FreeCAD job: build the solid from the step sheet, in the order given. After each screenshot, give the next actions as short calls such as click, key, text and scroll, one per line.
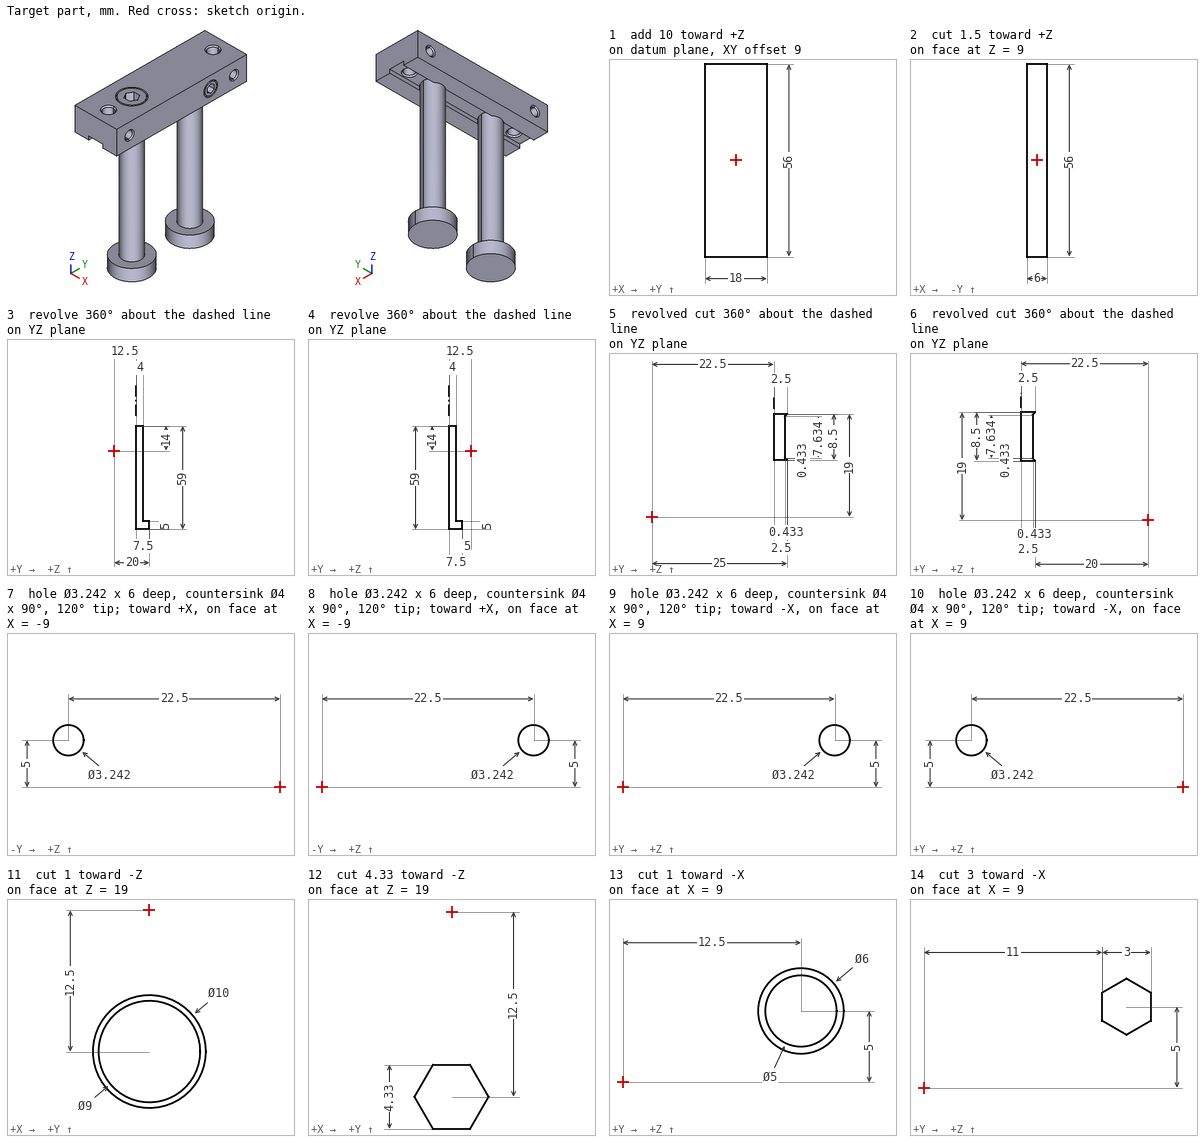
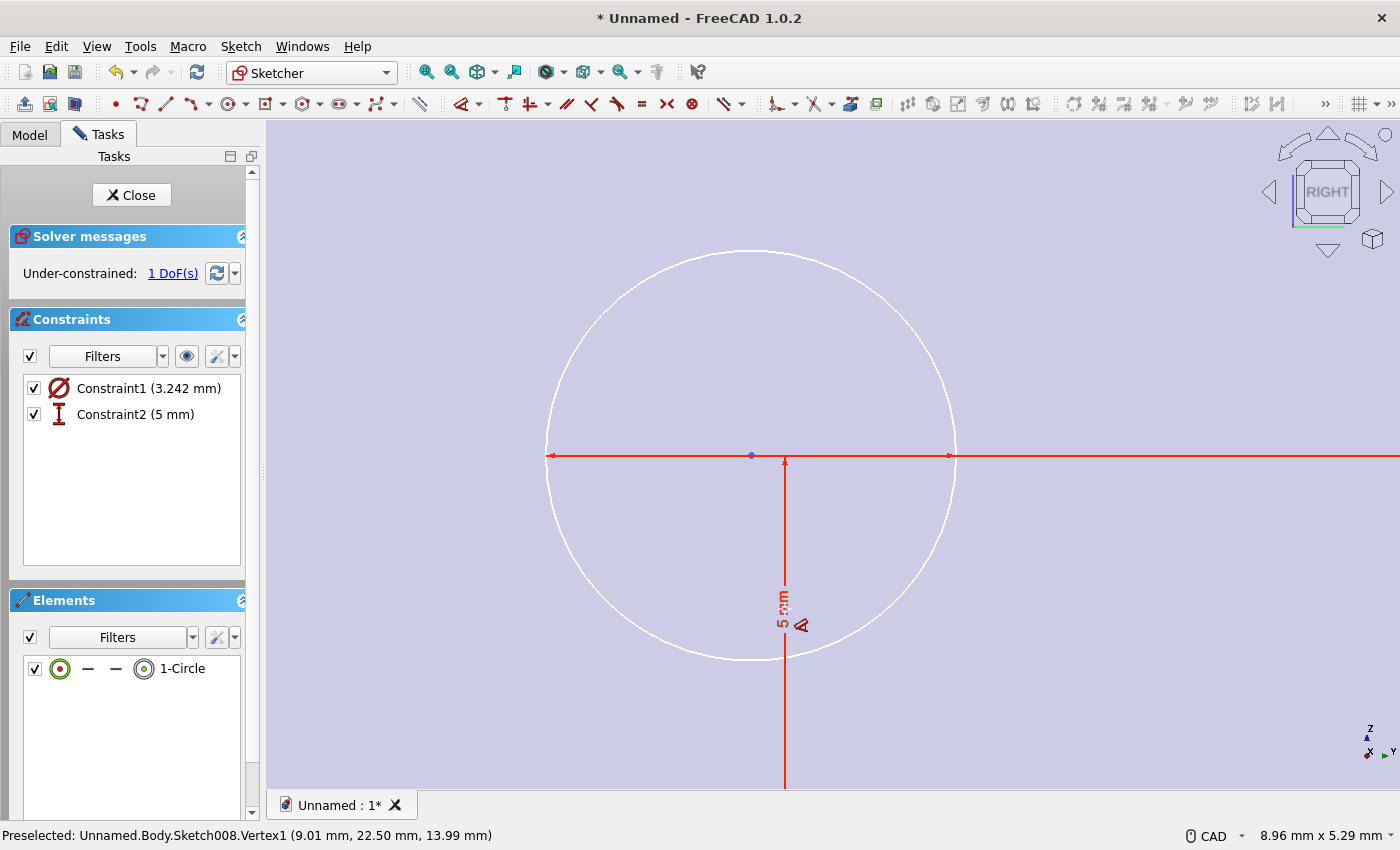
click(751, 456)
click(523, 422)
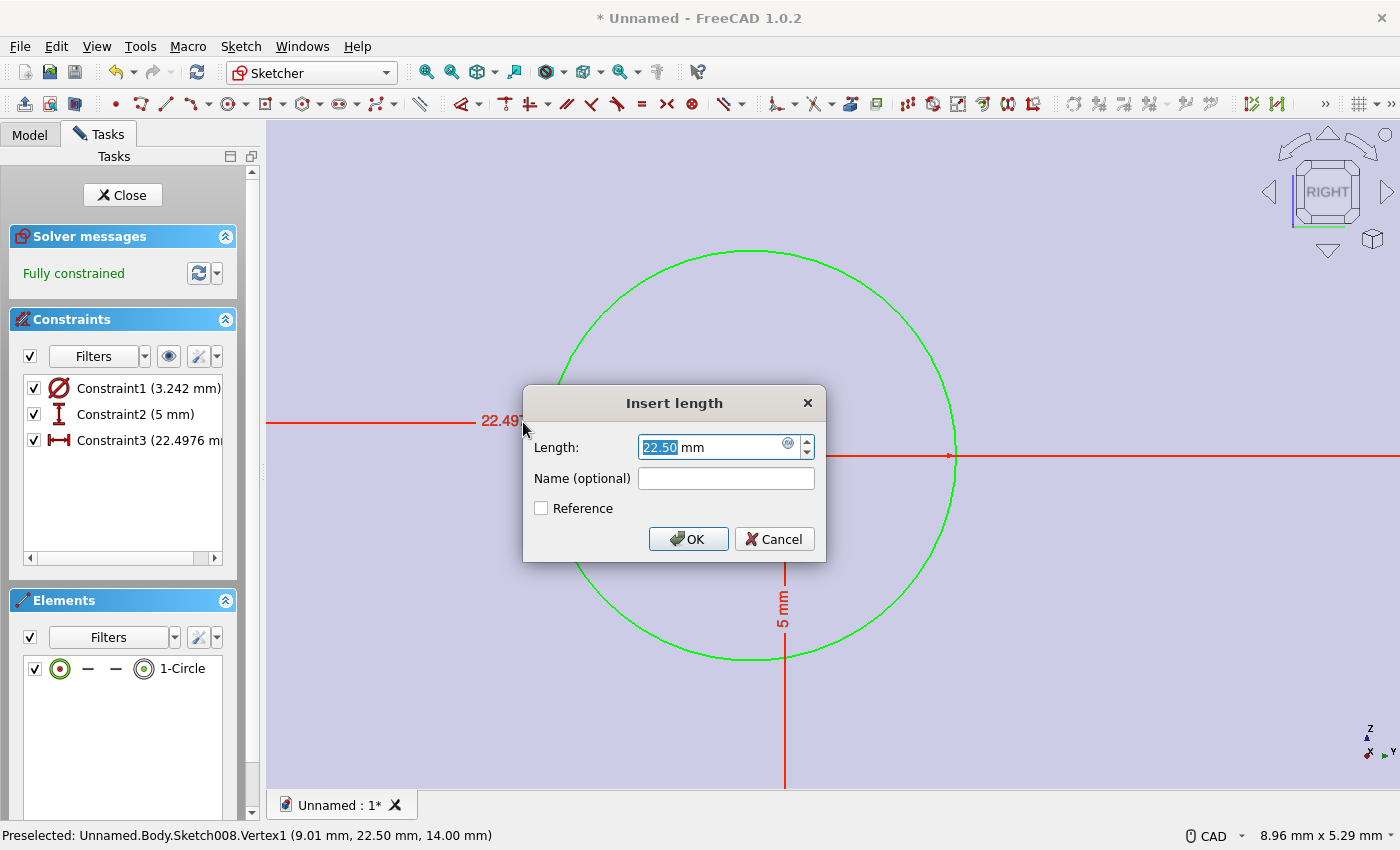
text(22.5)
key(Return)
key(Escape)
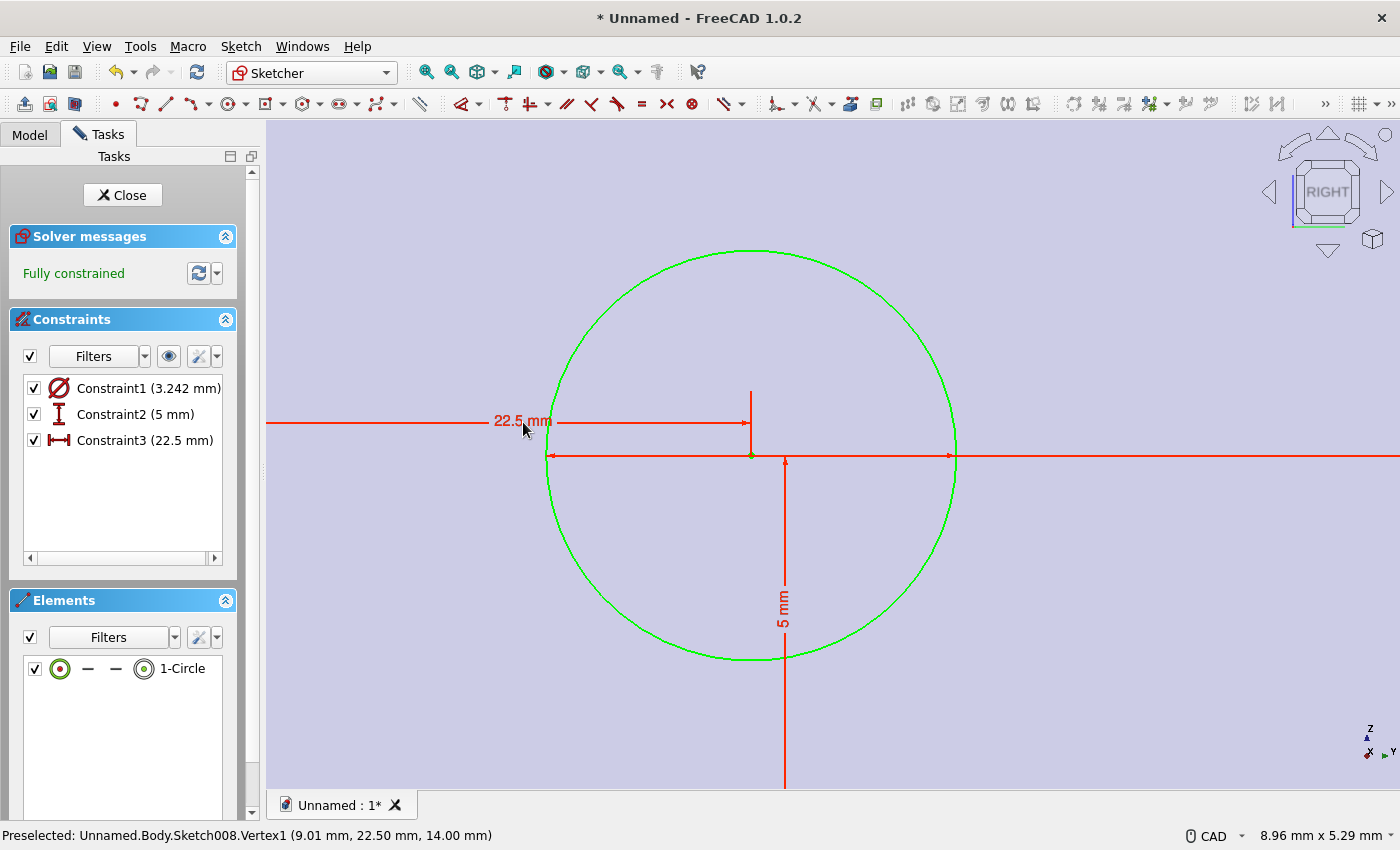
click(123, 195)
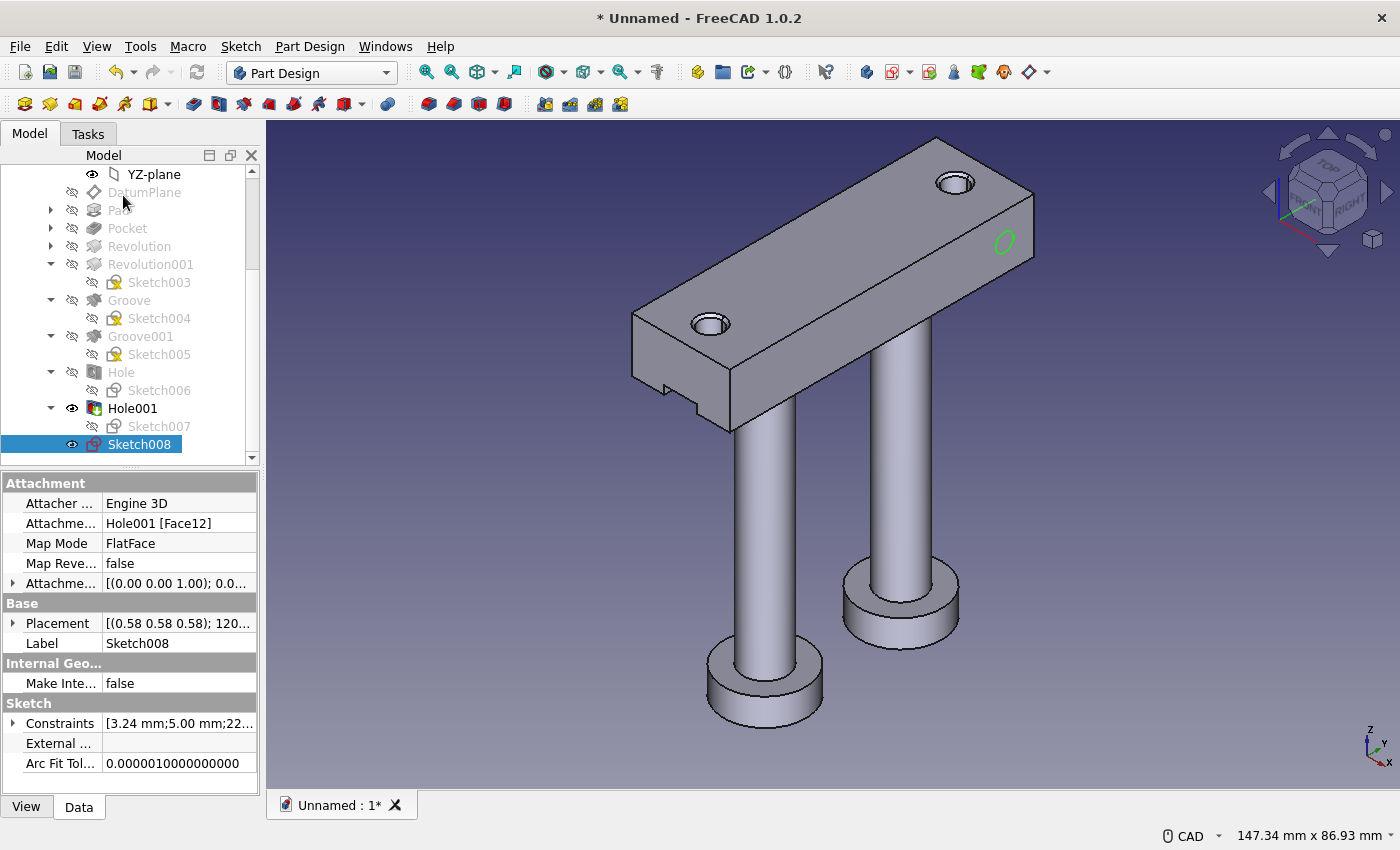
click(219, 104)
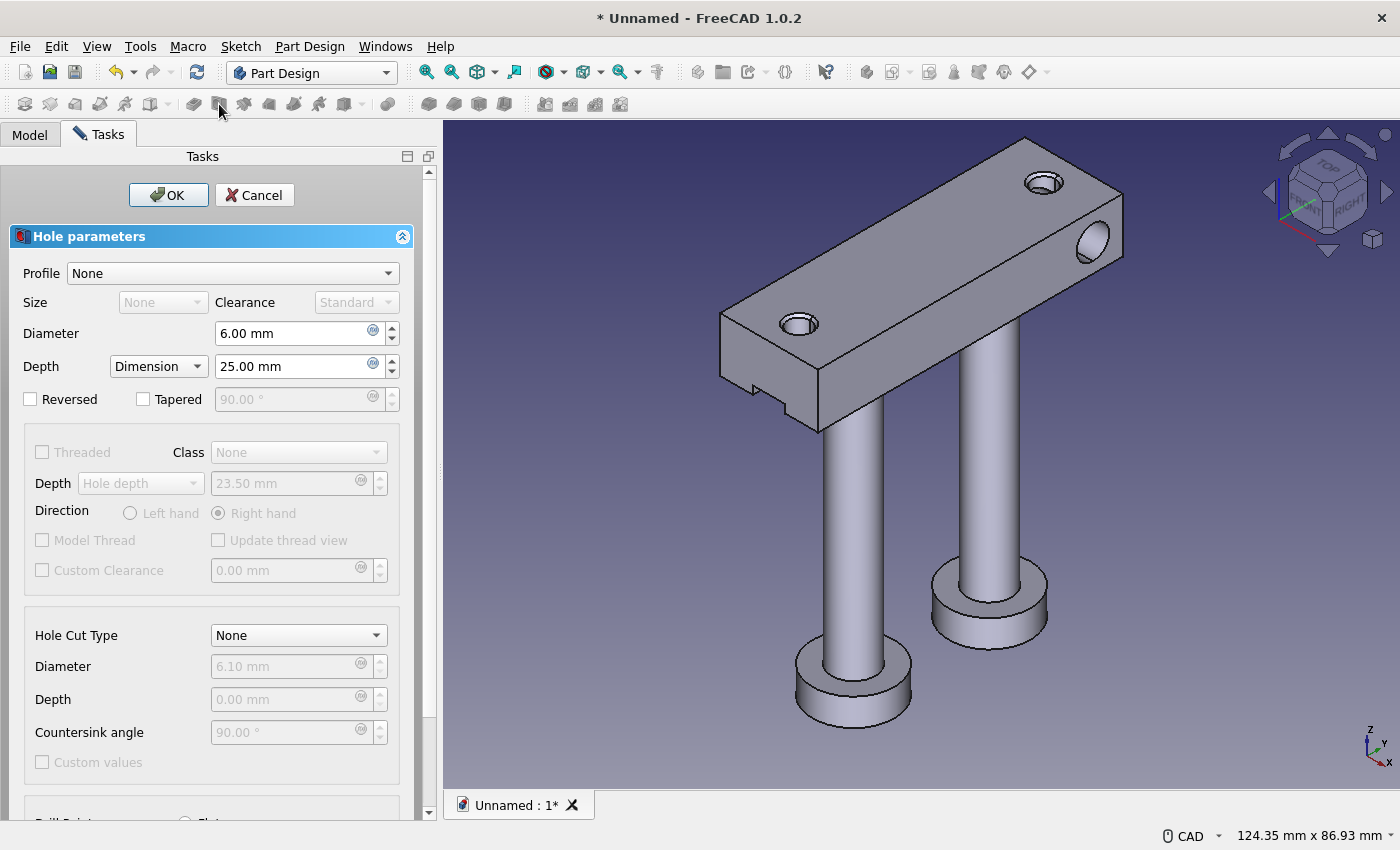
triple_click(300, 334)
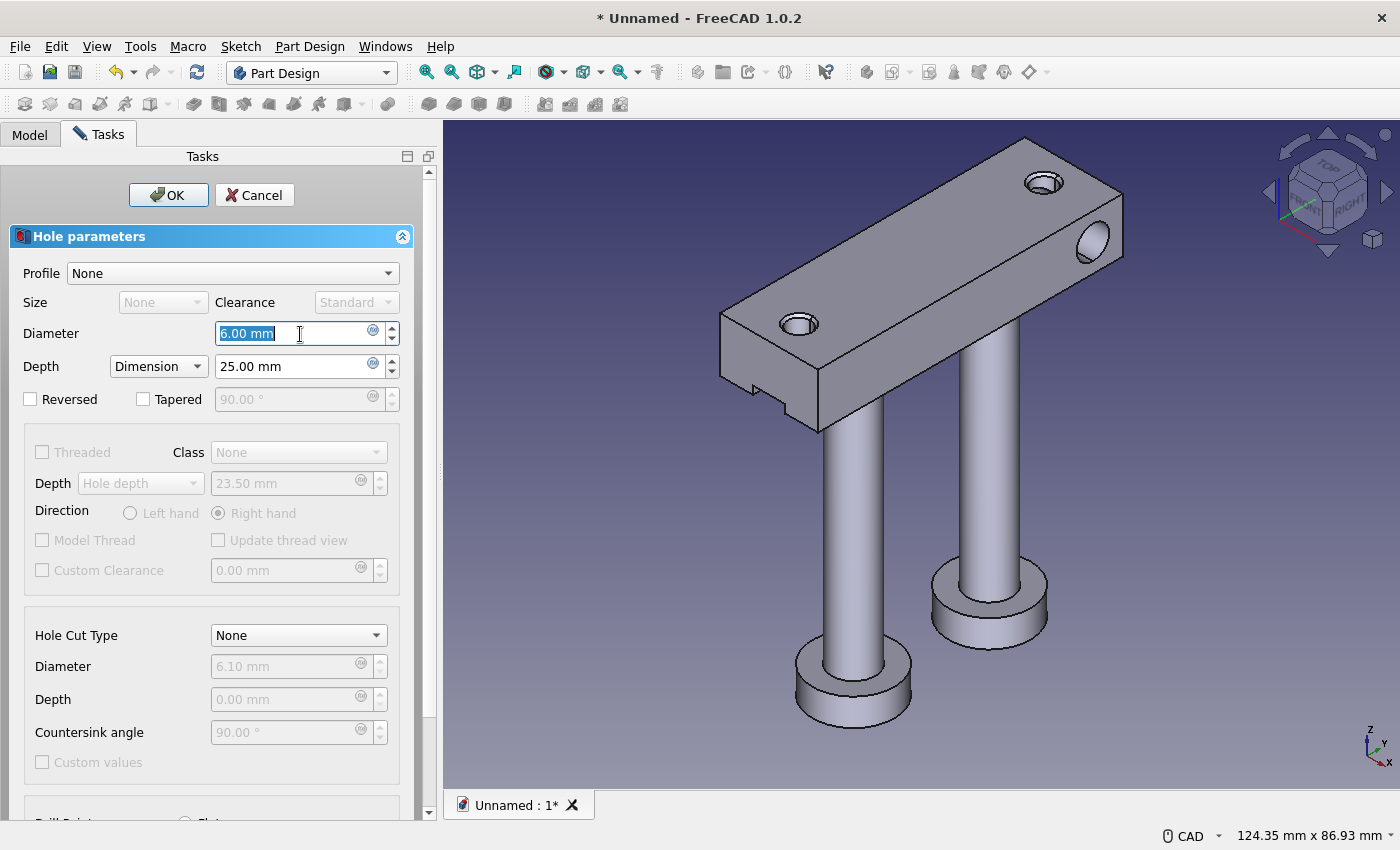
text(3.242)
key(Tab)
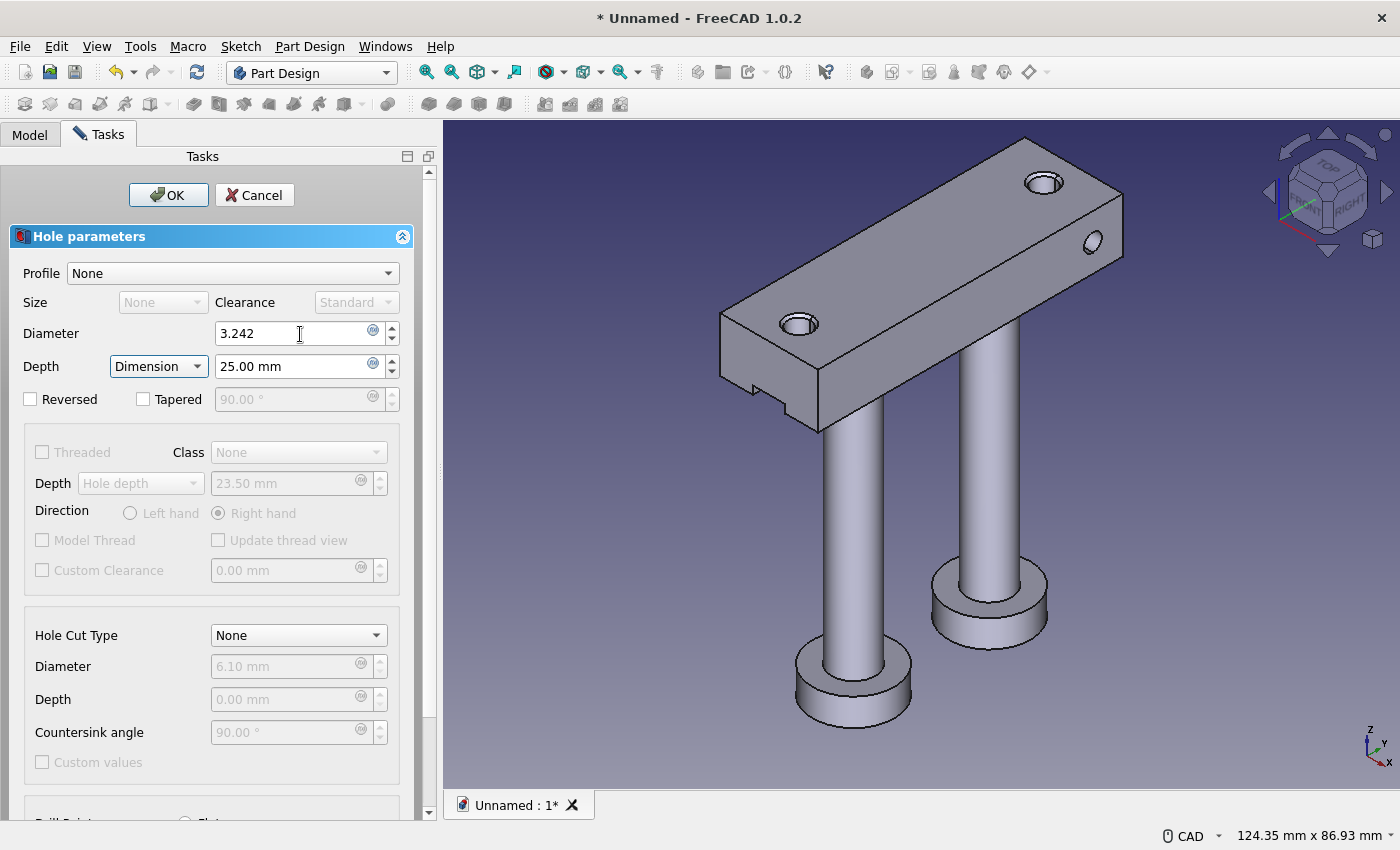
triple_click(300, 366)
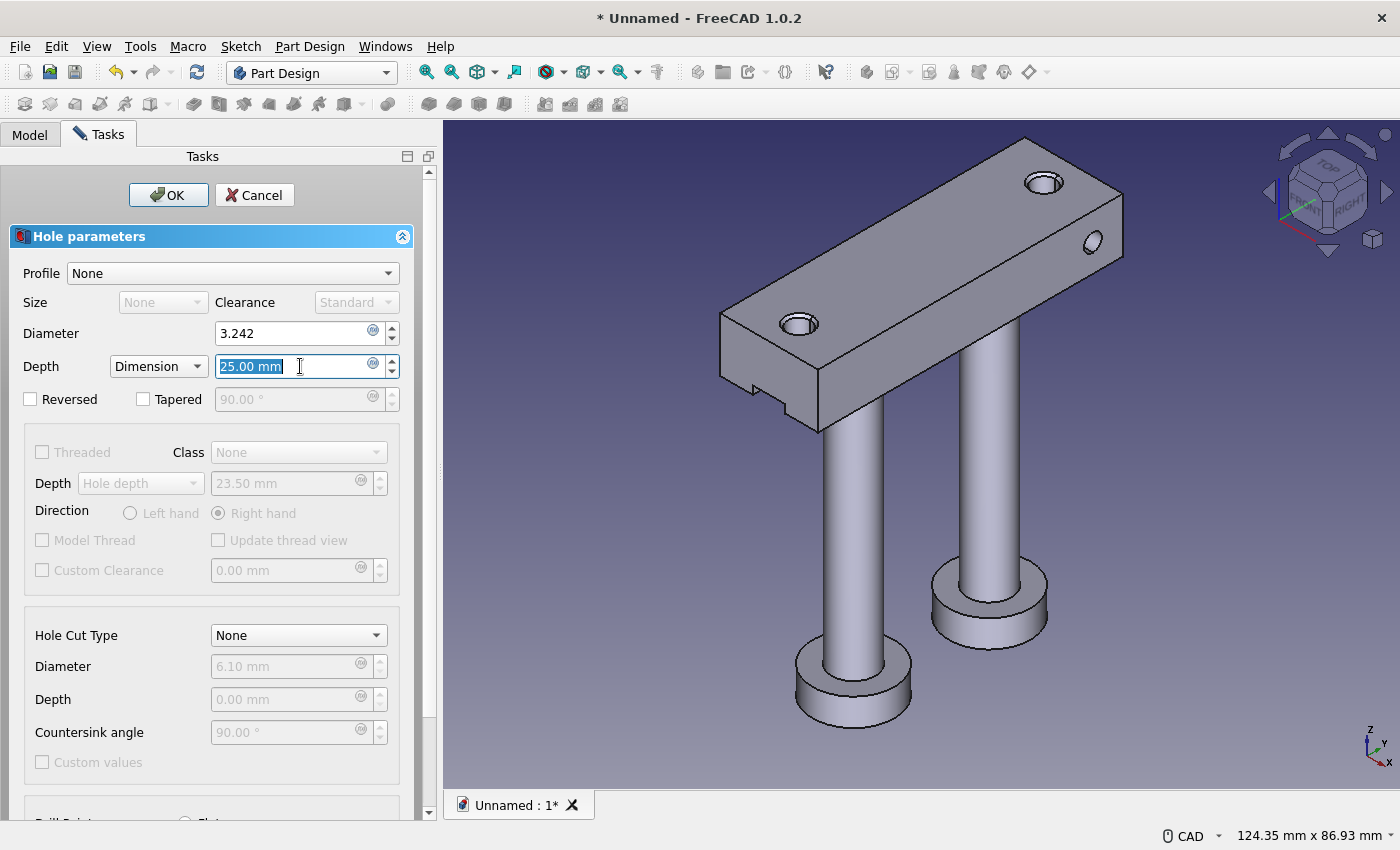
text(6)
key(Tab)